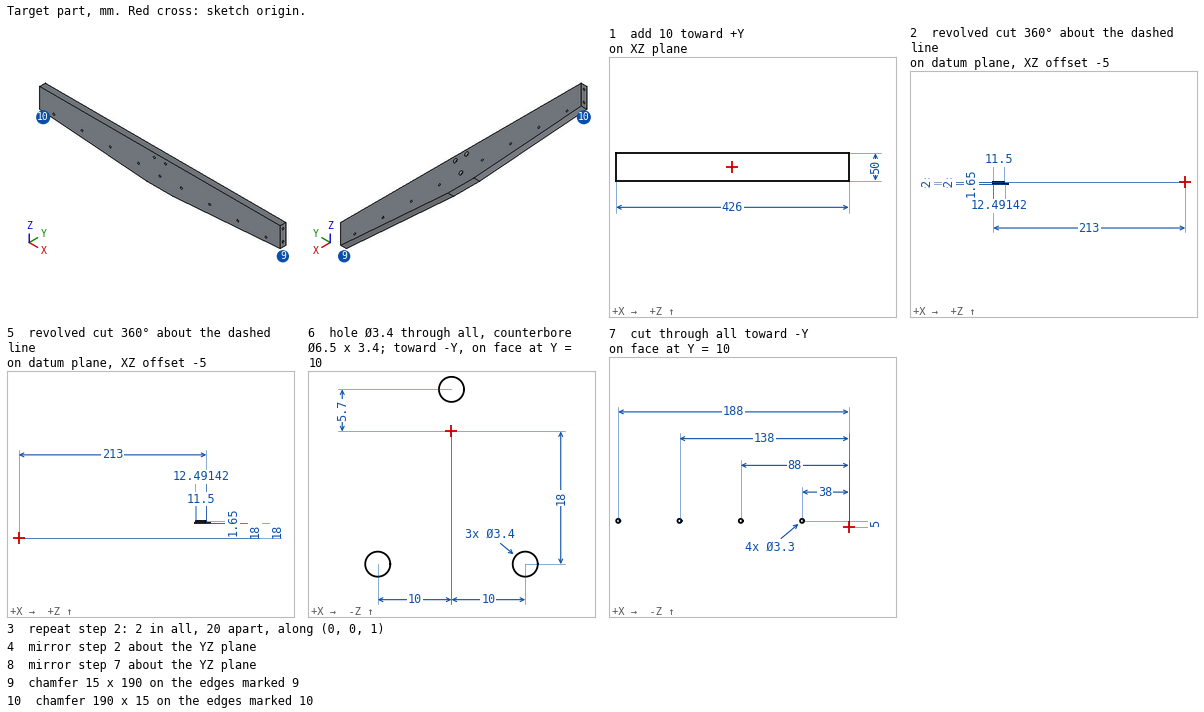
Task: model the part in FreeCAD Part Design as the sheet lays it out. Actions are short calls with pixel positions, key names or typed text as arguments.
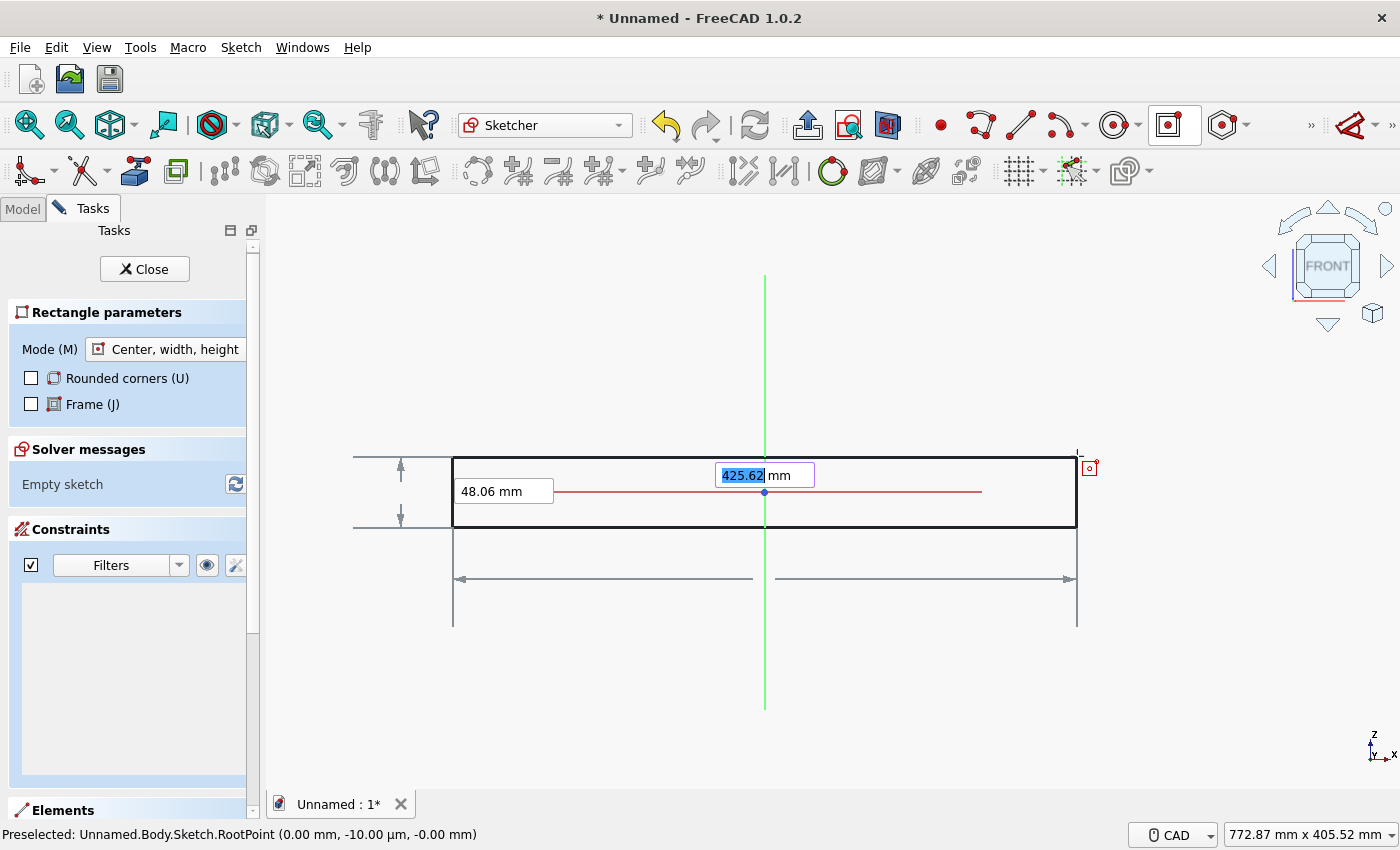
text(426)
key(Tab)
text(50)
key(Return)
key(Escape)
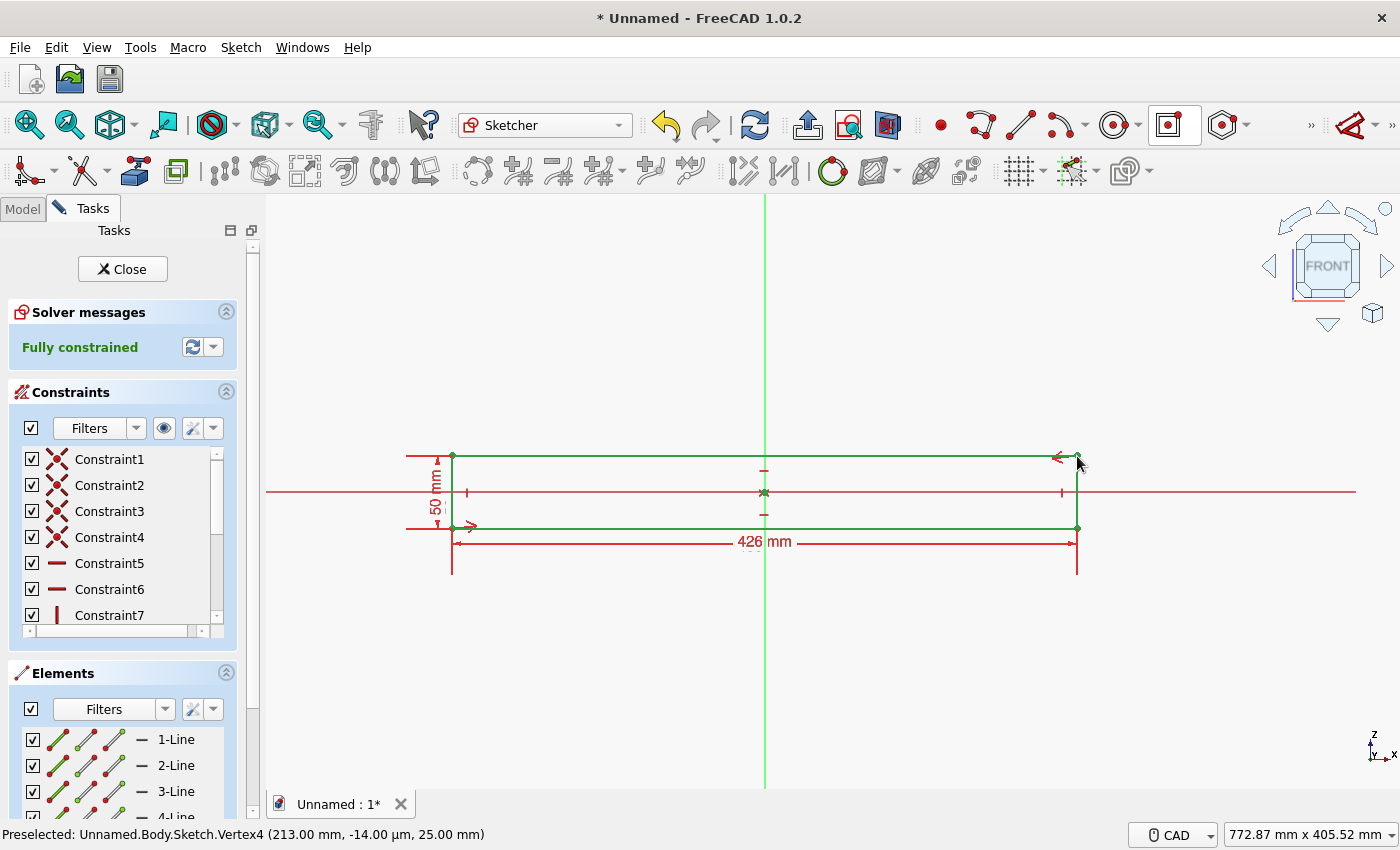
click(123, 269)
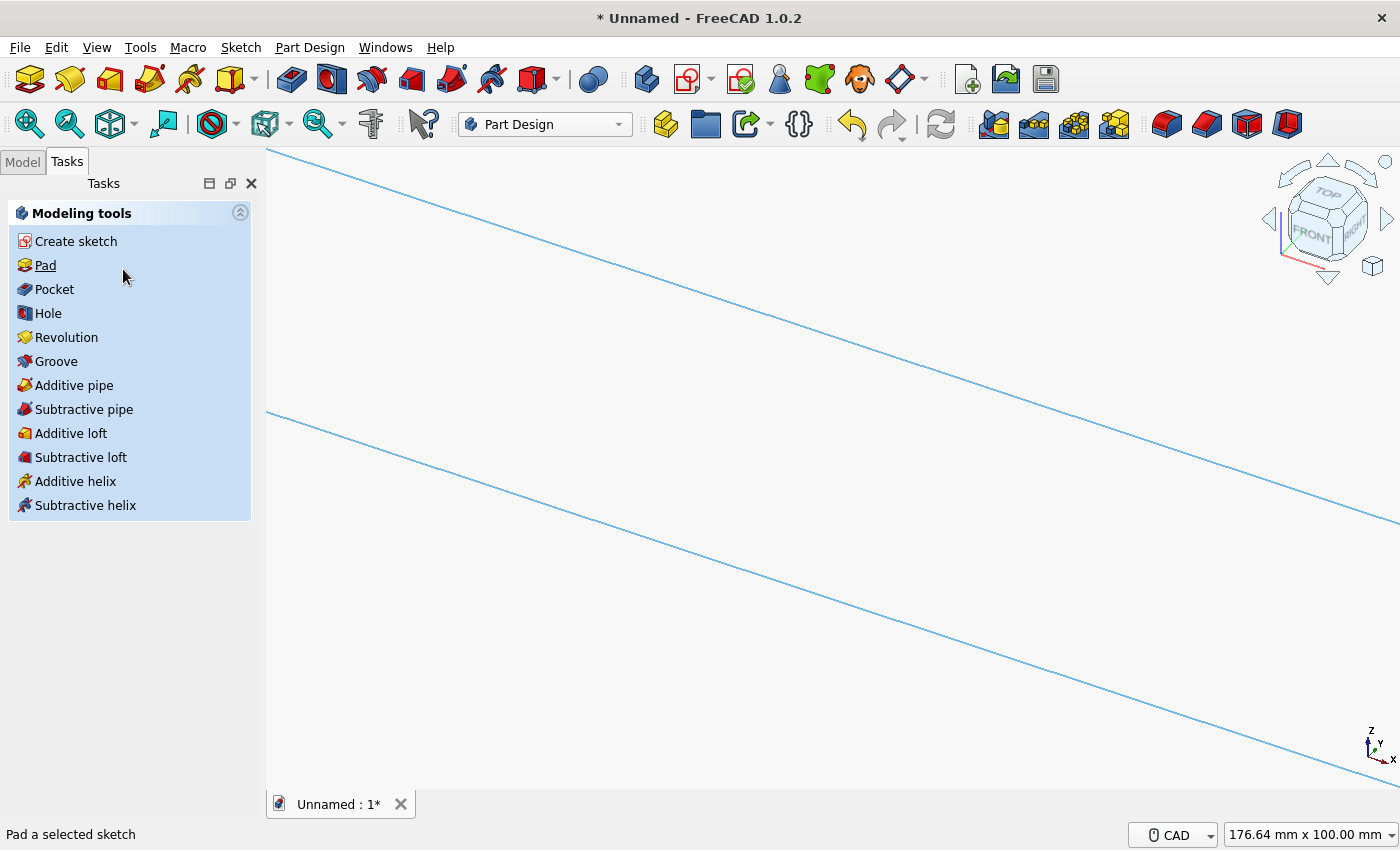
click(30, 80)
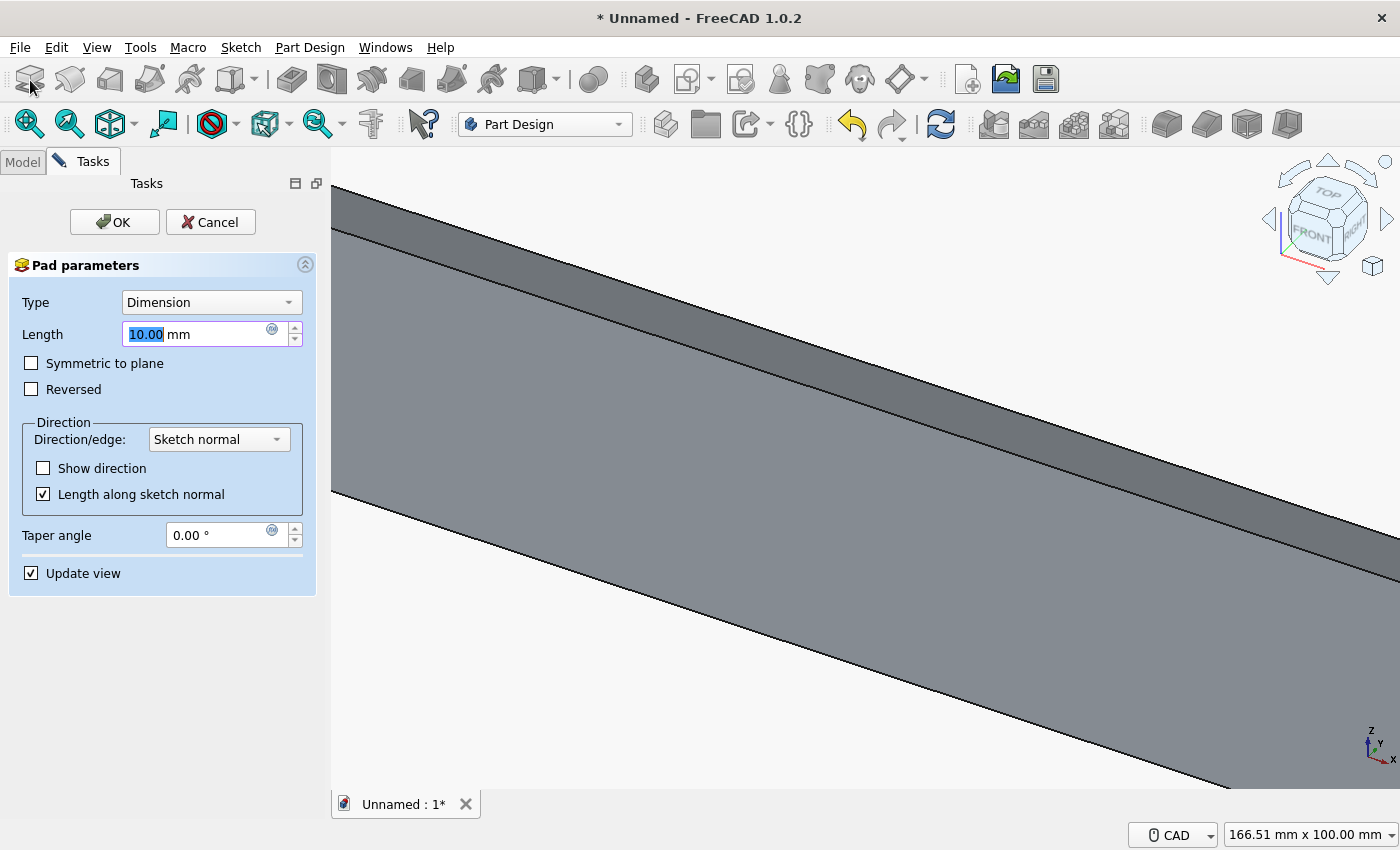
text(10)
key(Tab)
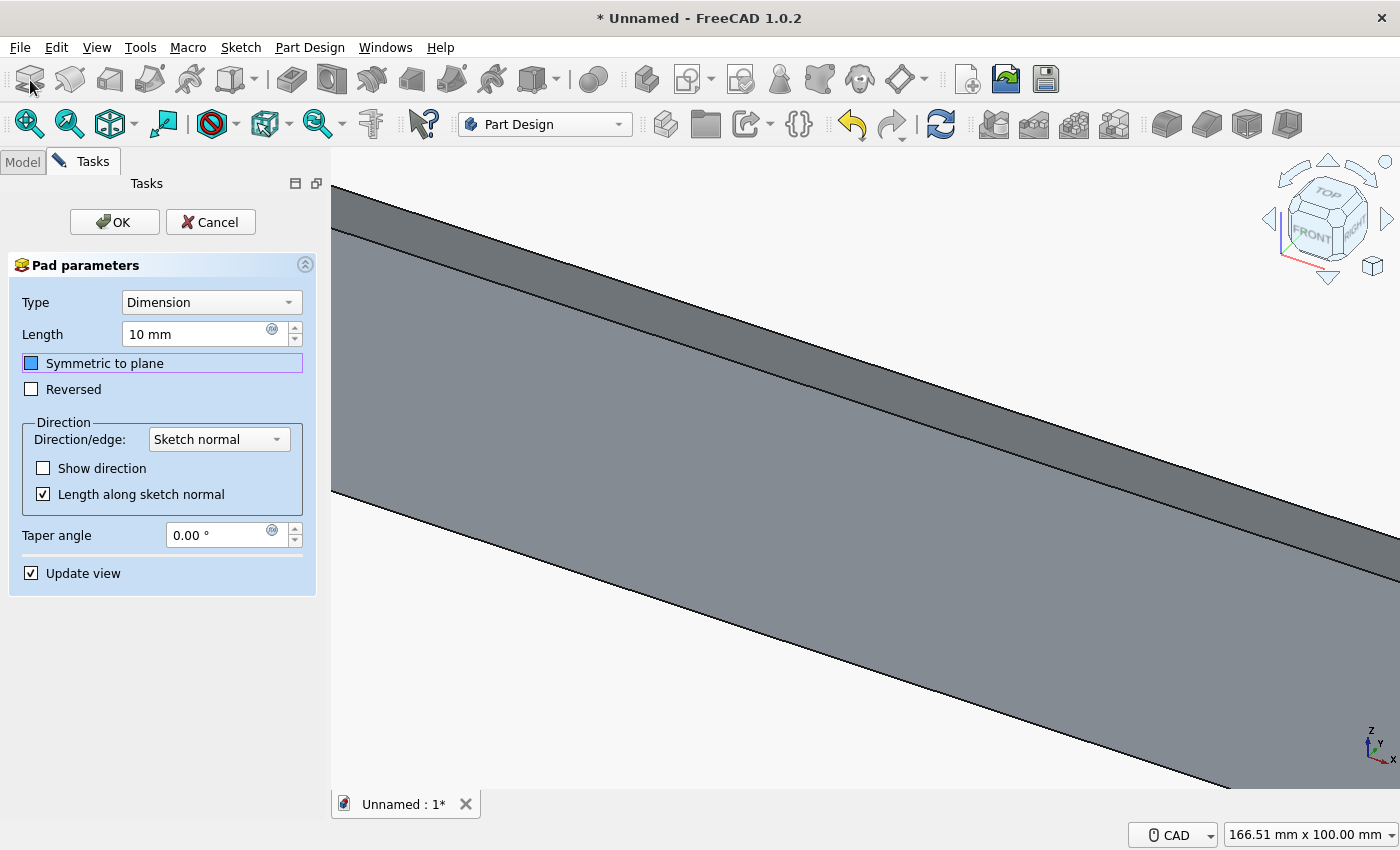
click(30, 389)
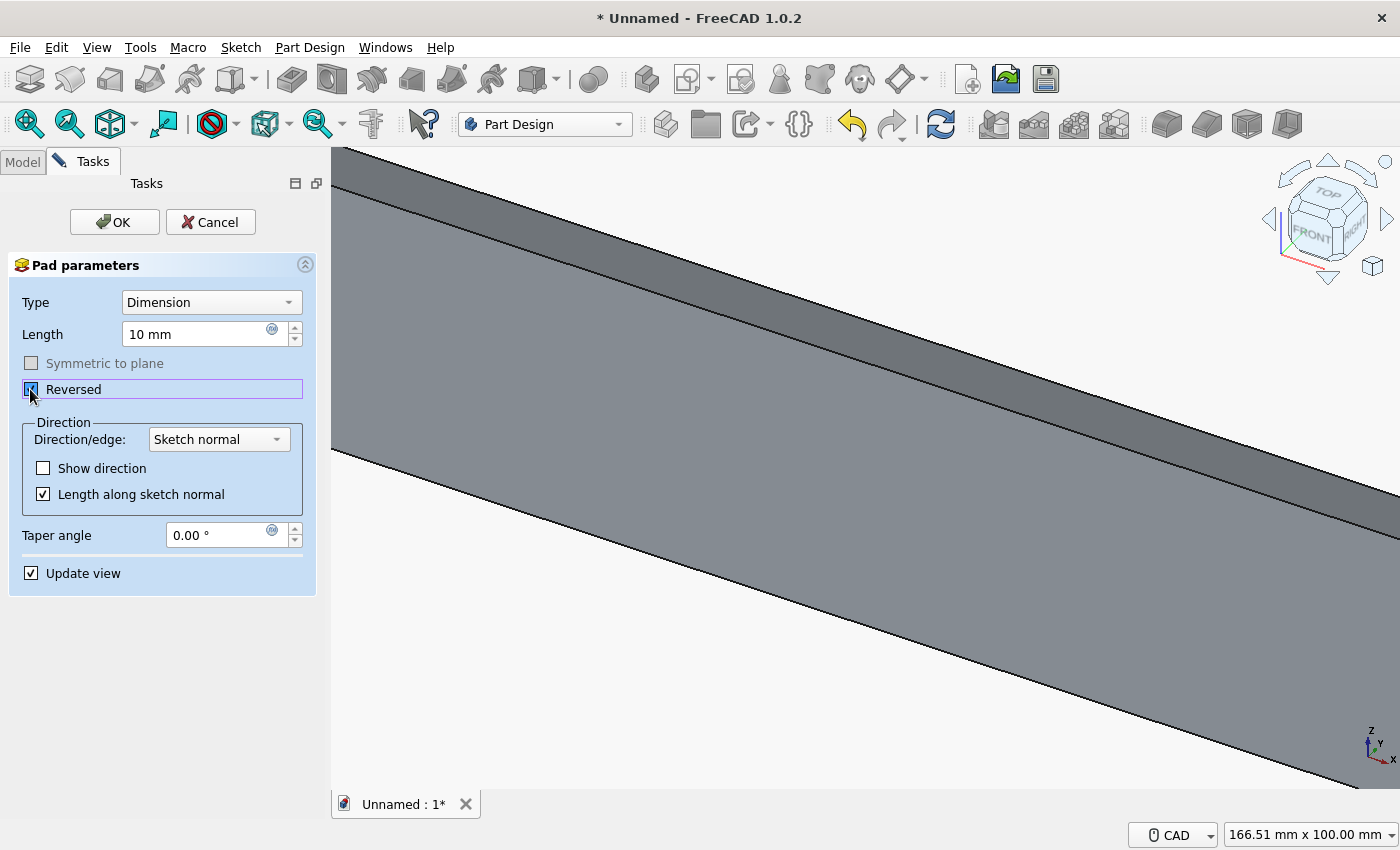
click(115, 222)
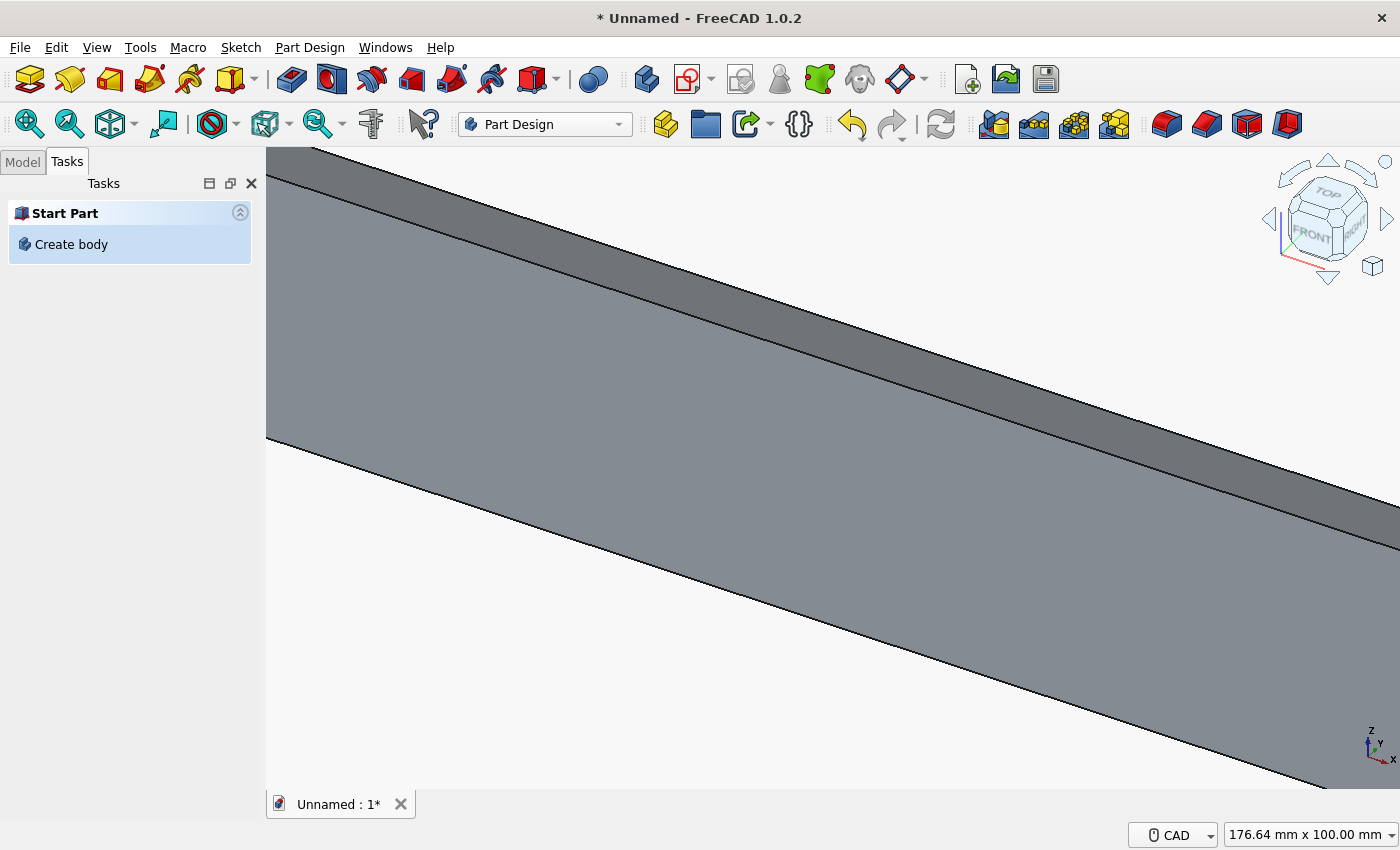
click(30, 124)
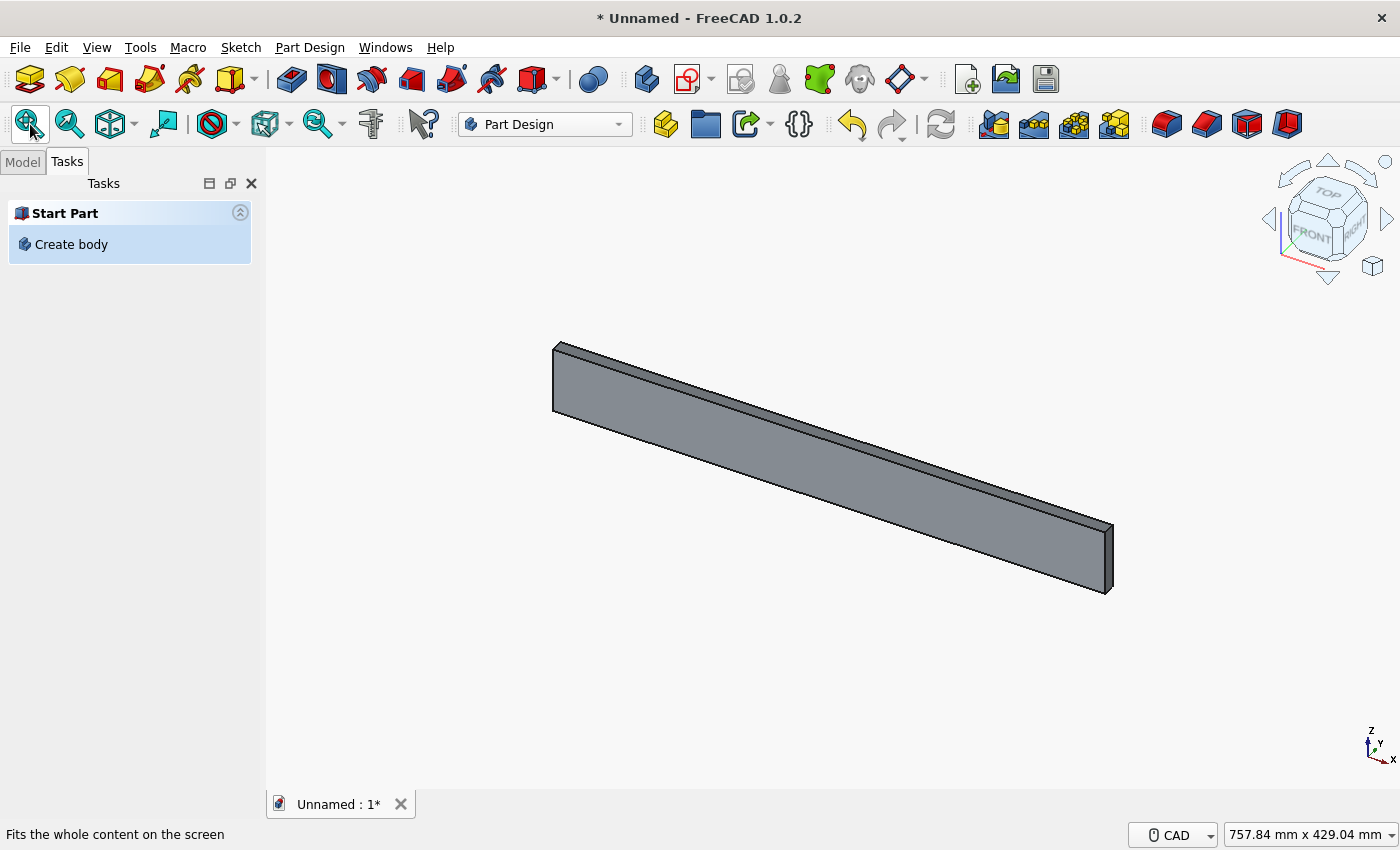
click(23, 161)